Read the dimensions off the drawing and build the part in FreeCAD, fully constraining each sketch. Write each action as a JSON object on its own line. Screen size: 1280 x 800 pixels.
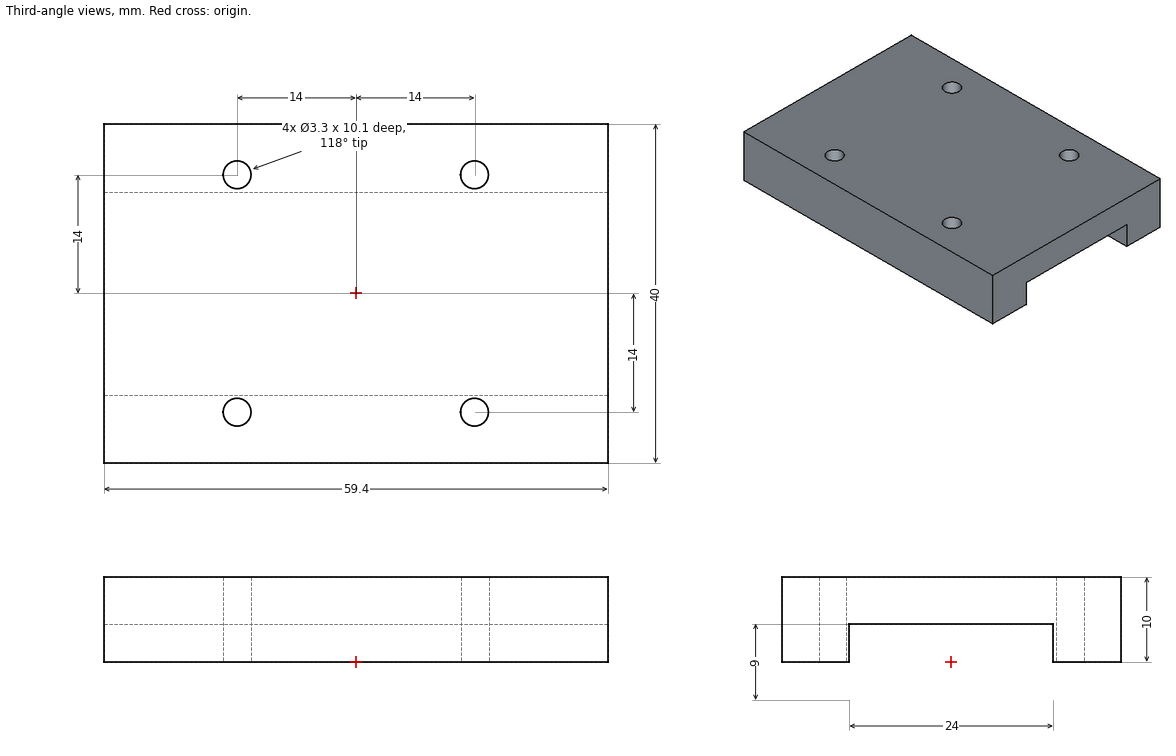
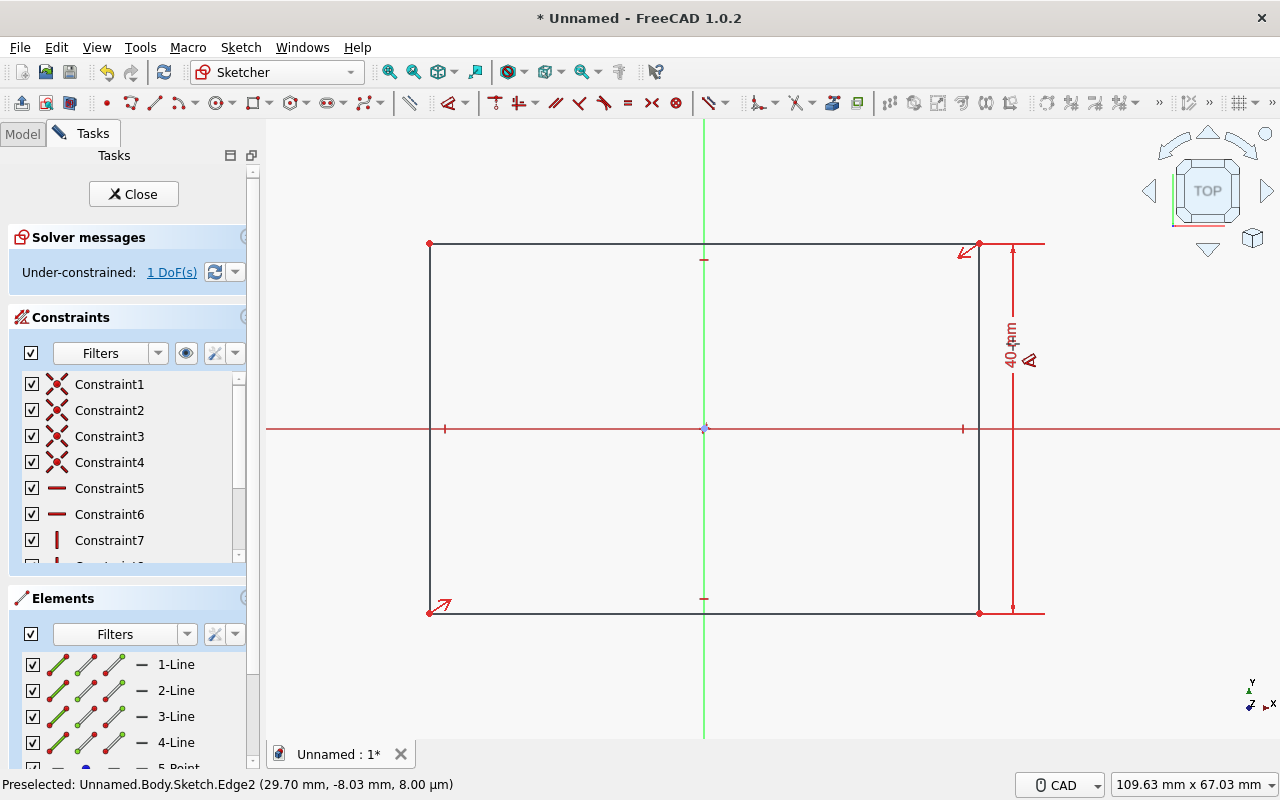
{"action": "left_click", "coordinate": [594, 614]}
{"action": "left_click", "coordinate": [578, 648]}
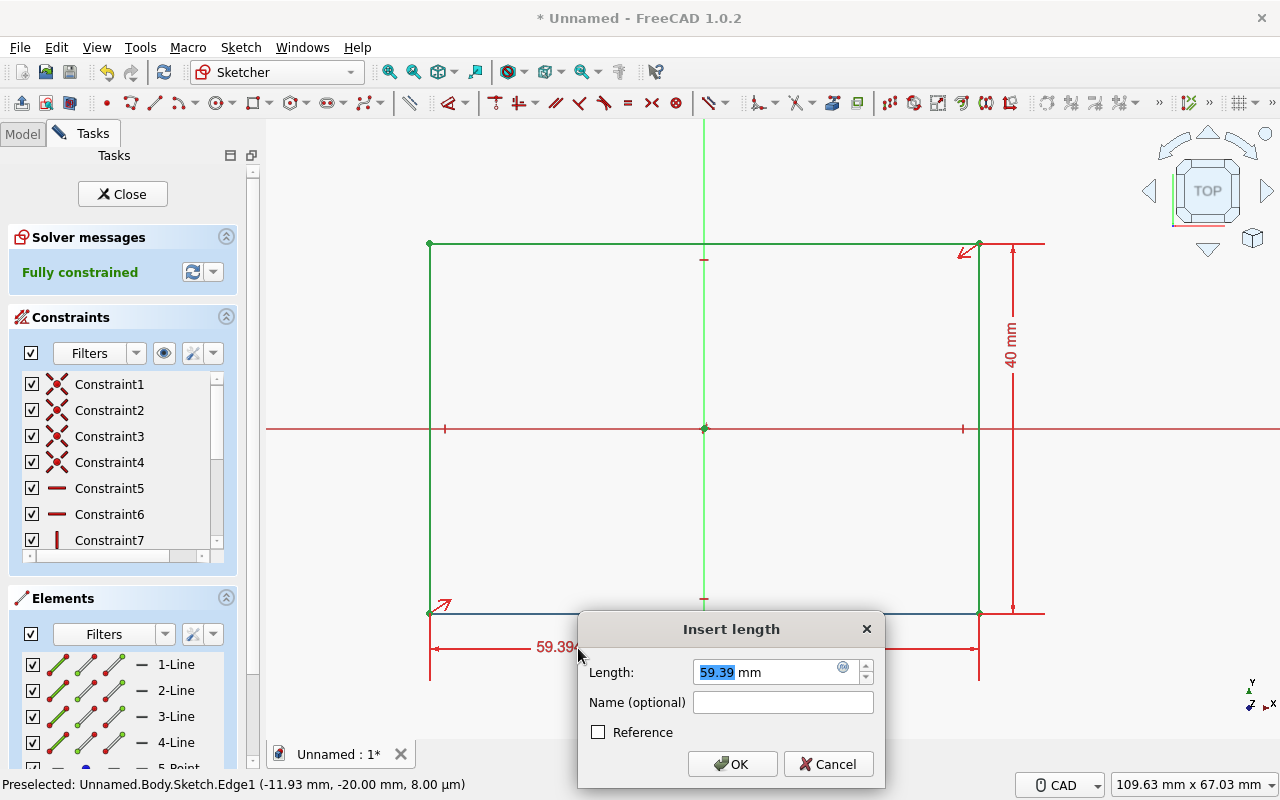
{"action": "type", "text": "59.4"}
{"action": "key", "text": "Return"}
{"action": "key", "text": "Escape"}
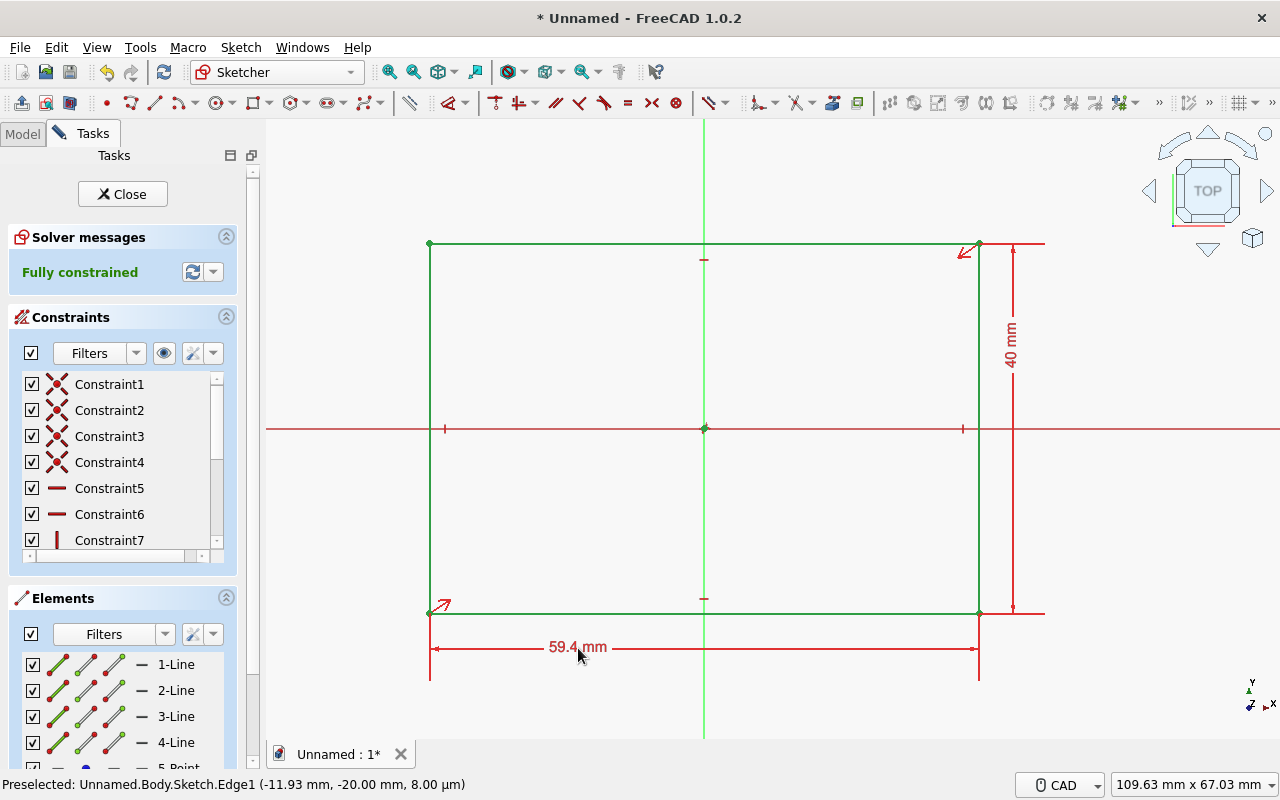
{"action": "left_click", "coordinate": [123, 194]}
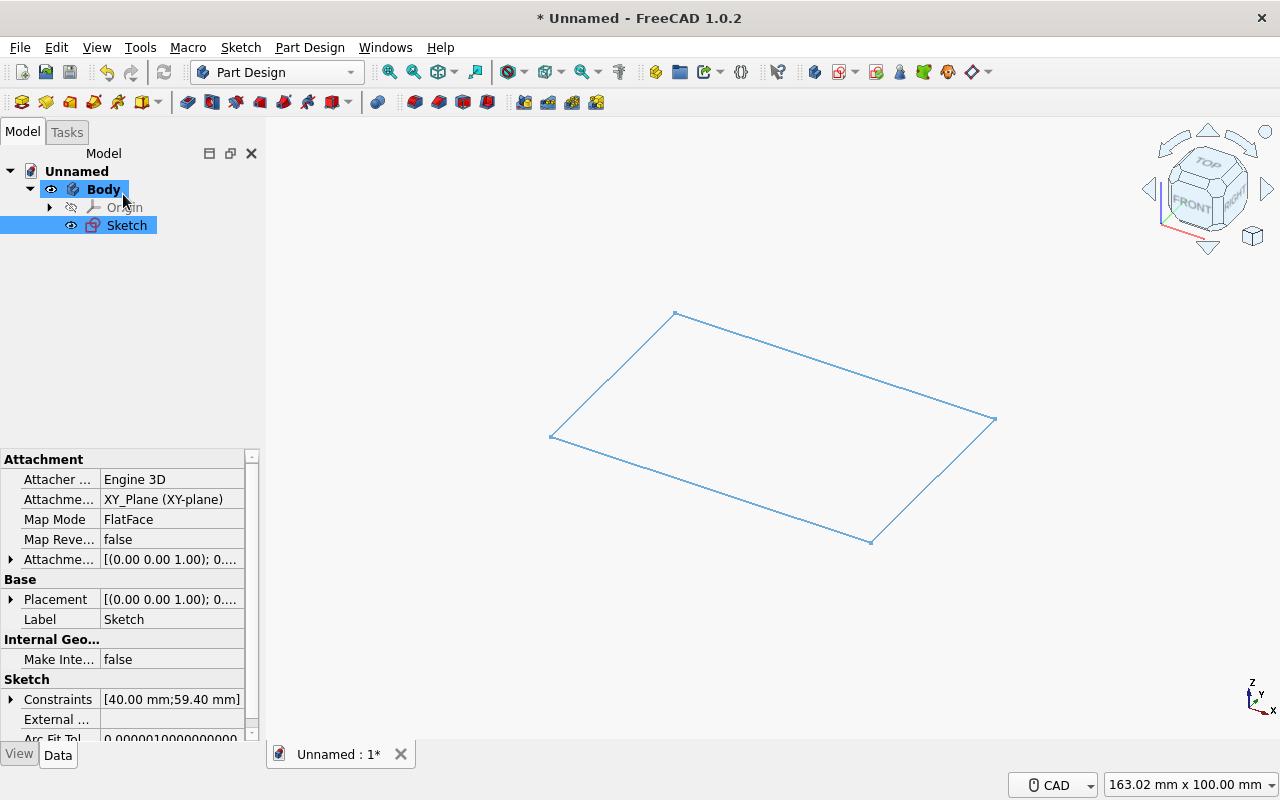
{"action": "left_click", "coordinate": [22, 102]}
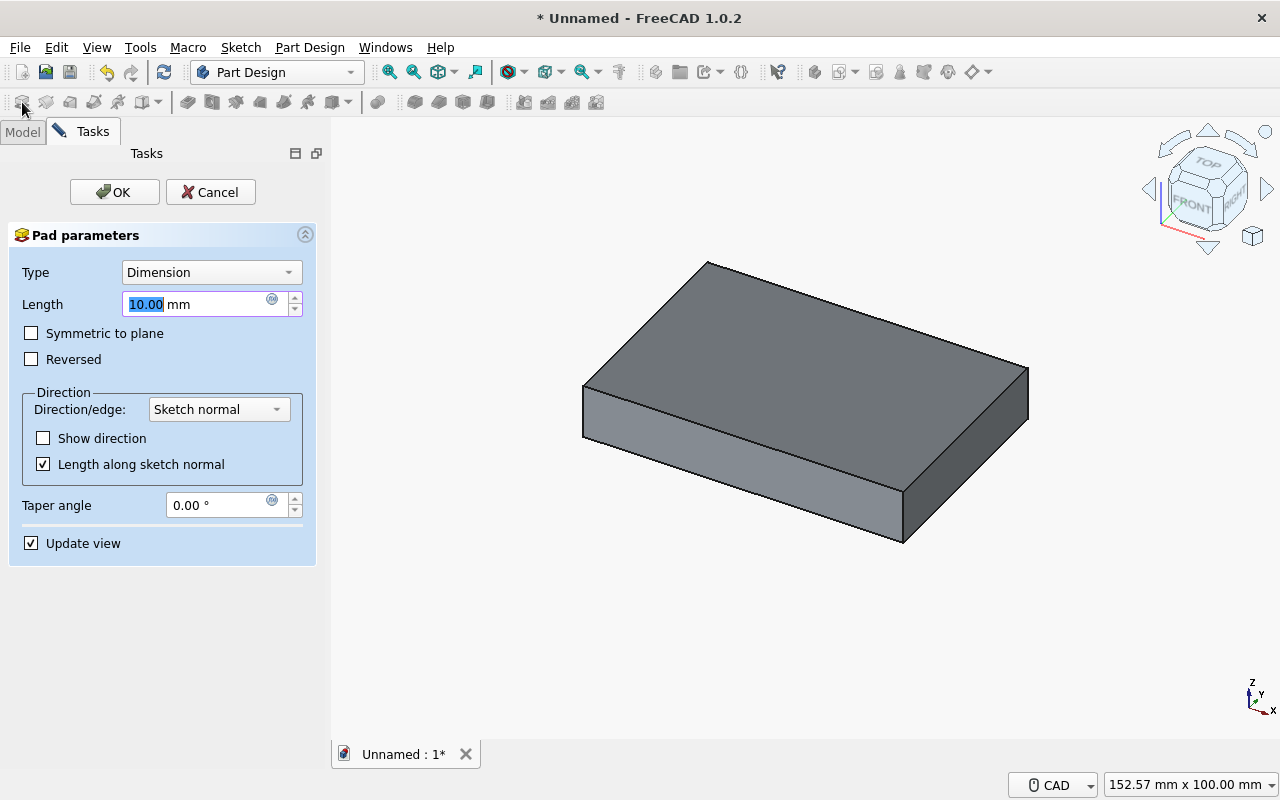
{"action": "type", "text": "10"}
{"action": "key", "text": "Tab"}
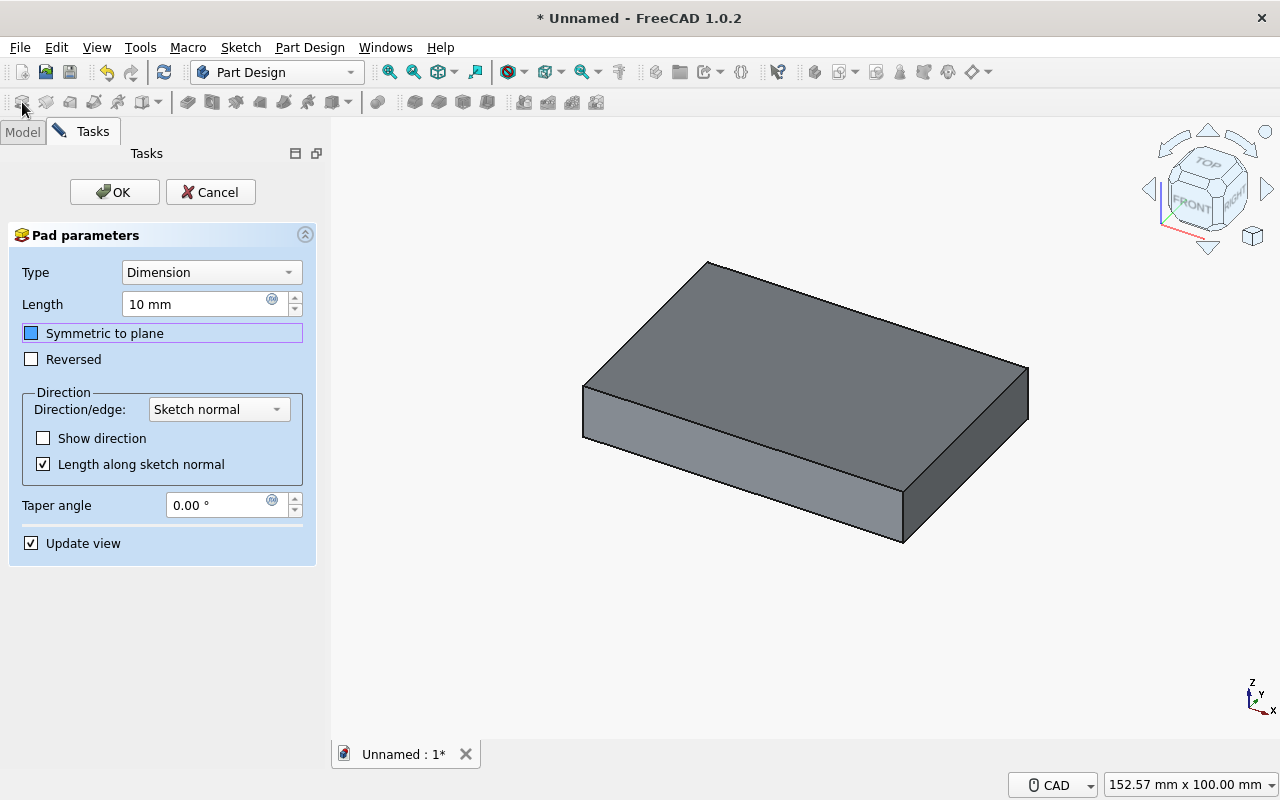
{"action": "left_click", "coordinate": [115, 192]}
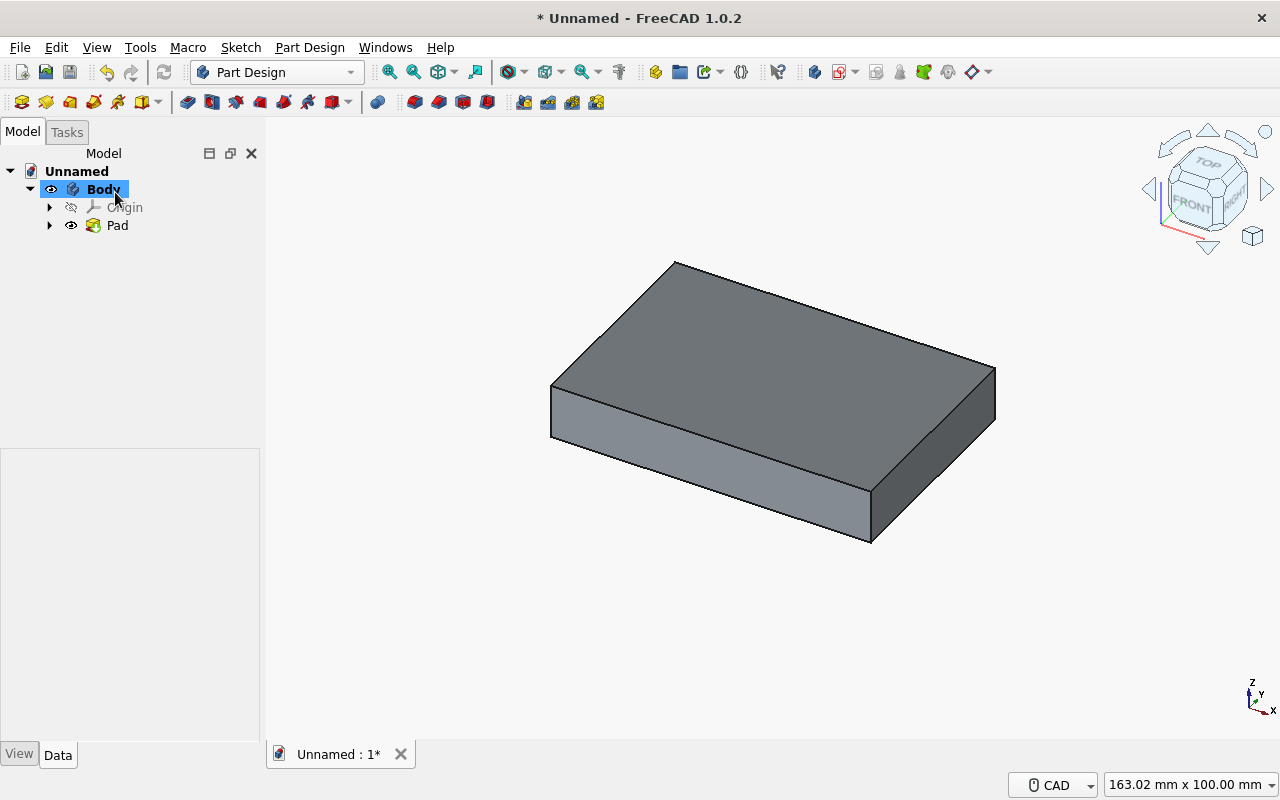
{"action": "key", "text": "6"}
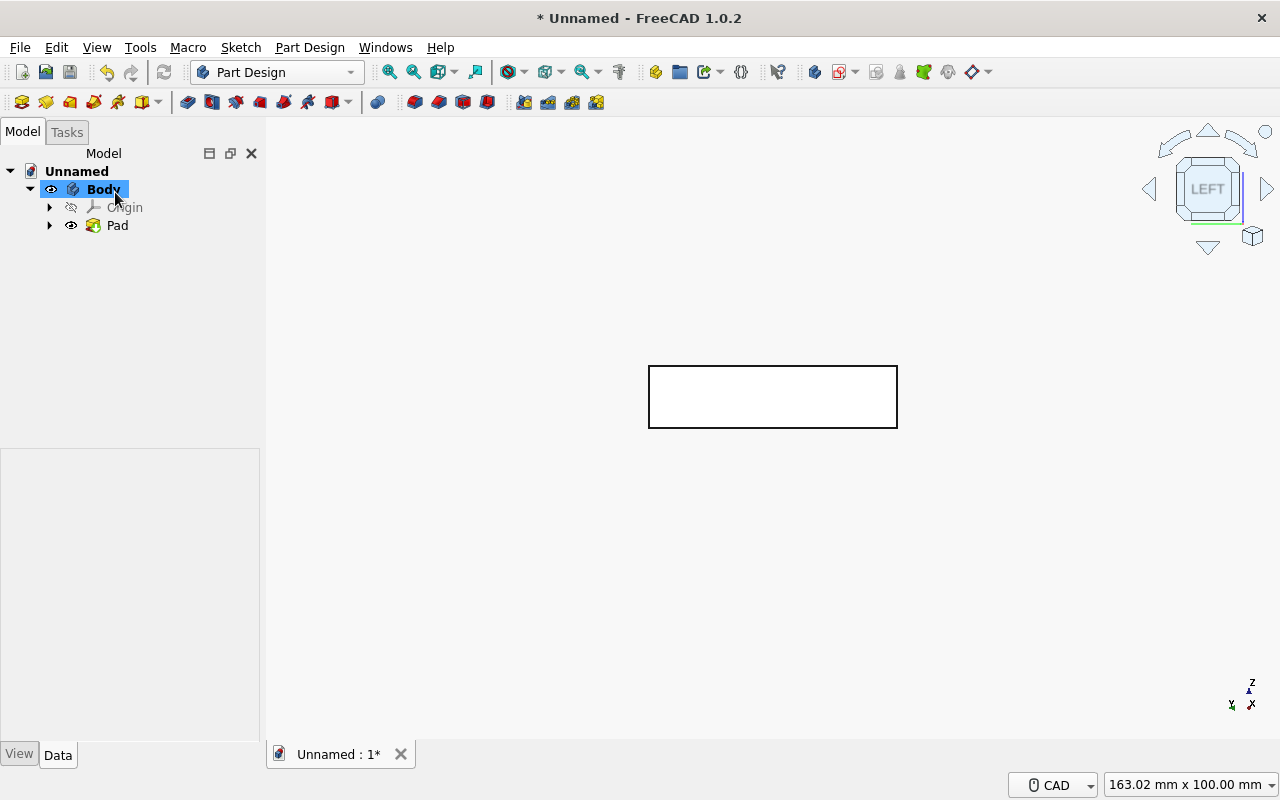
{"action": "key", "text": "v f"}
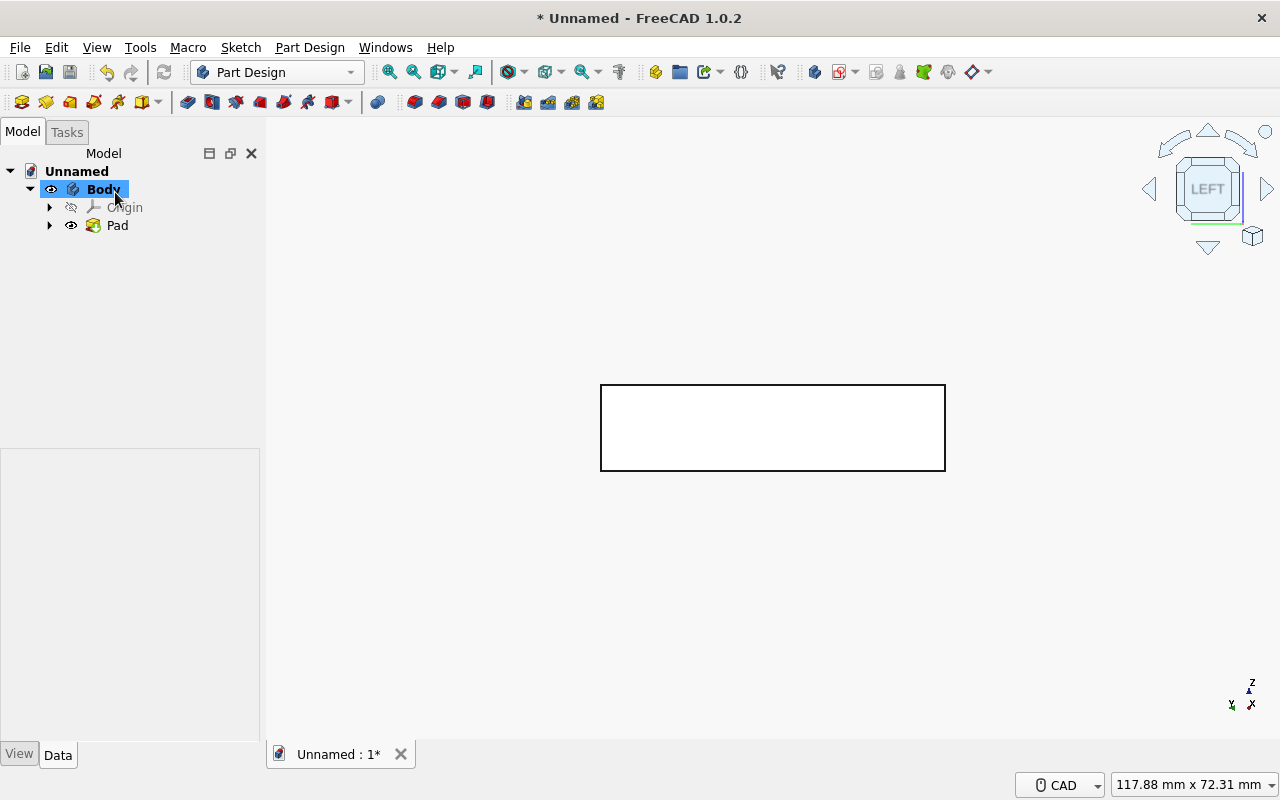
{"action": "left_click", "coordinate": [675, 427]}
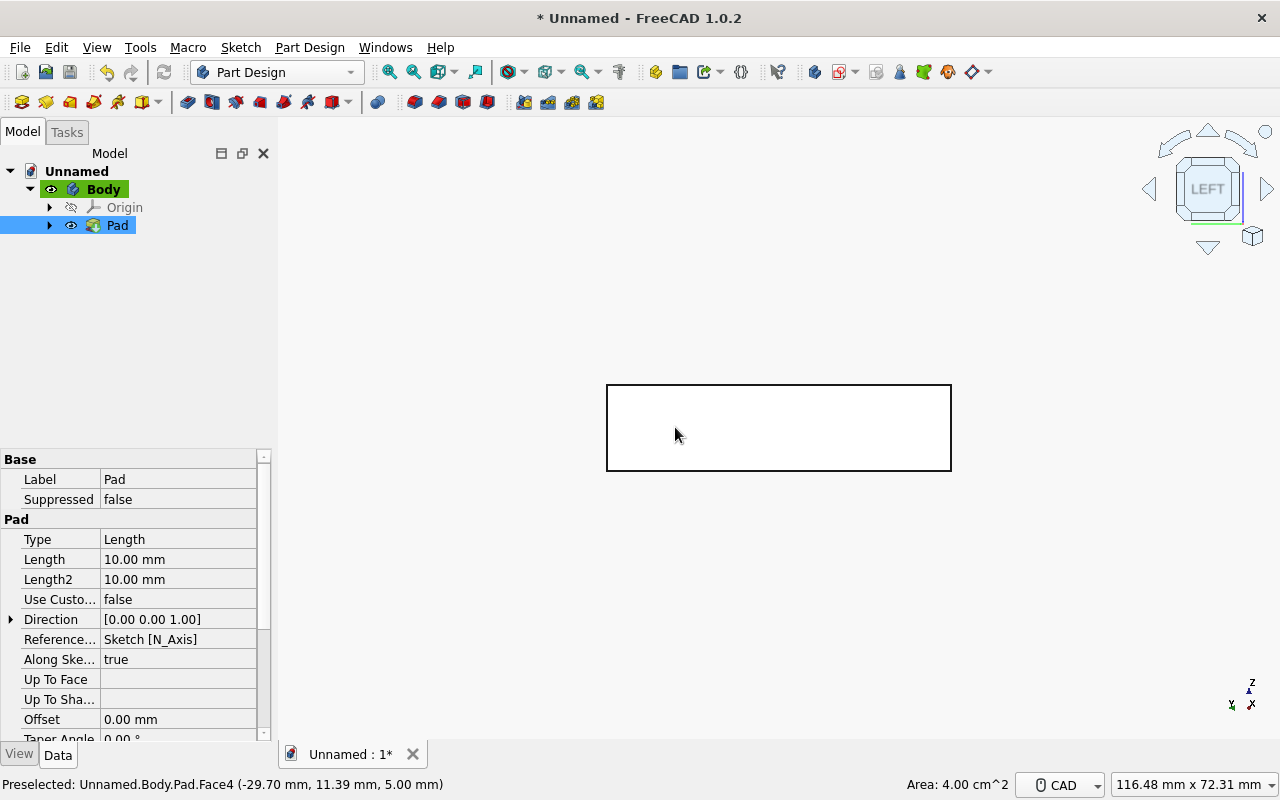
{"action": "left_click", "coordinate": [840, 72]}